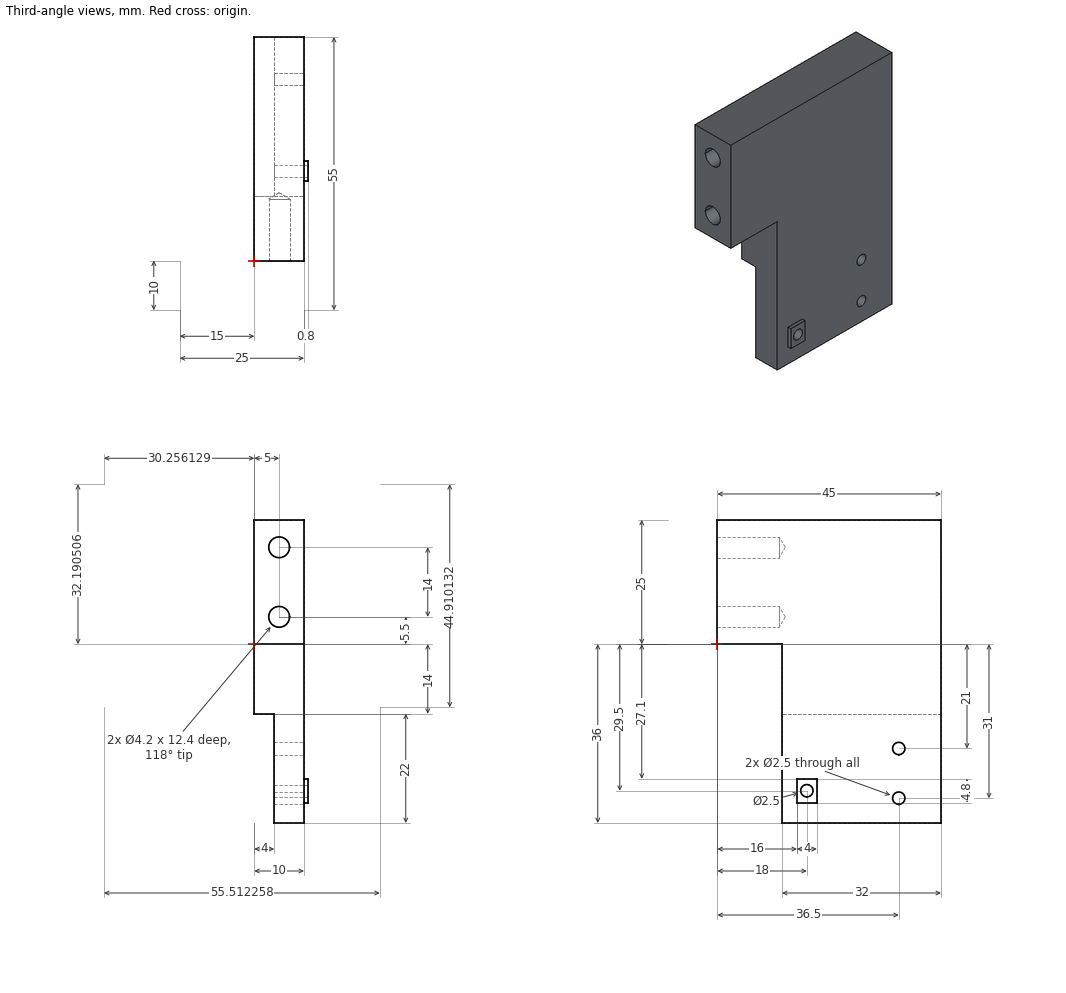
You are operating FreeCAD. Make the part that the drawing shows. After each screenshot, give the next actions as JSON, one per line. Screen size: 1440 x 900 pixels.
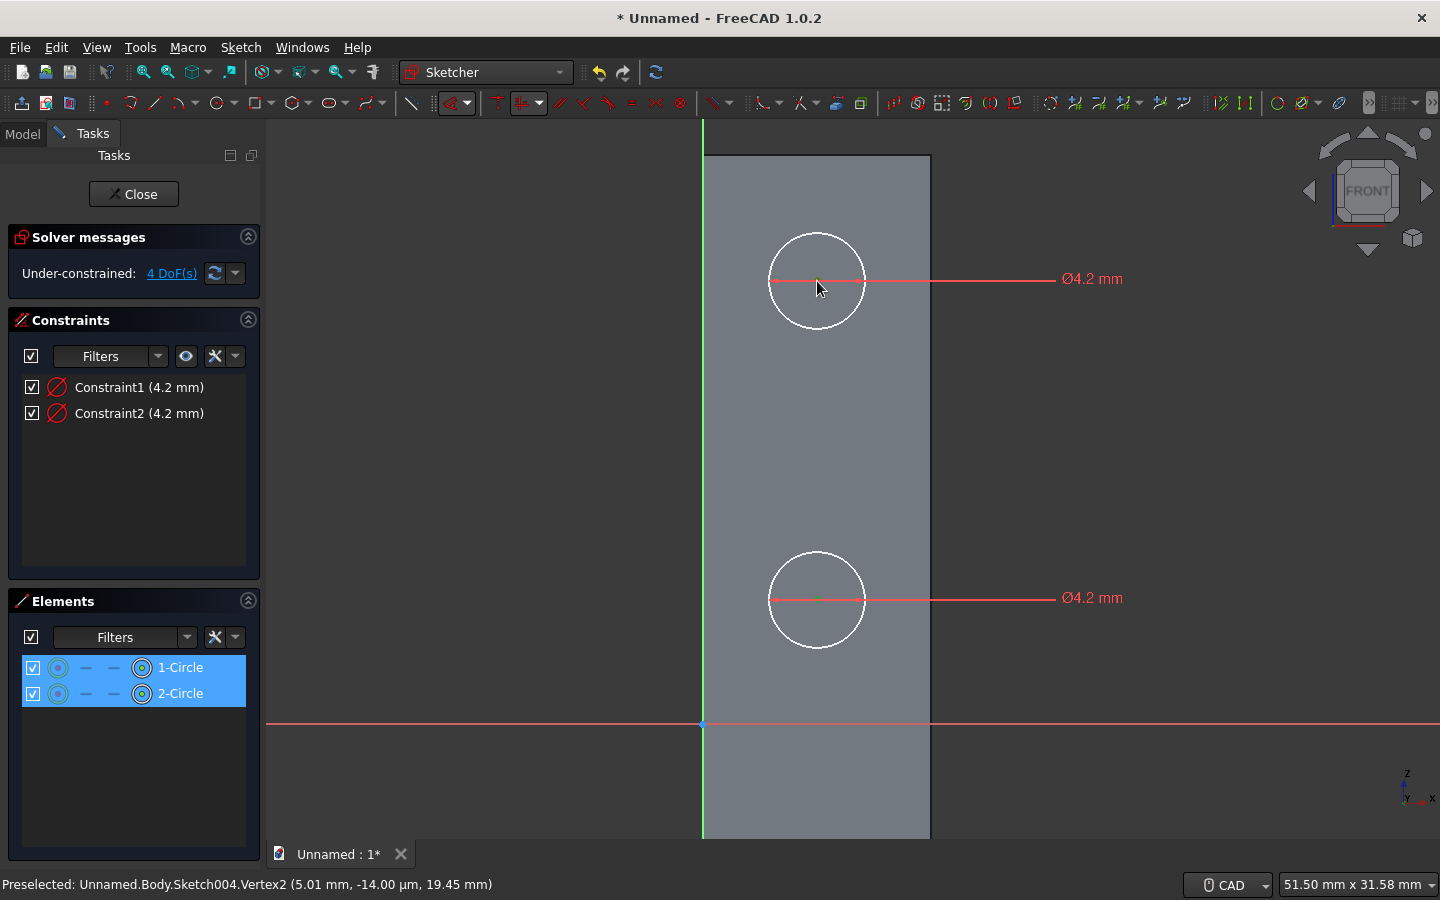
{"action": "key", "text": "v"}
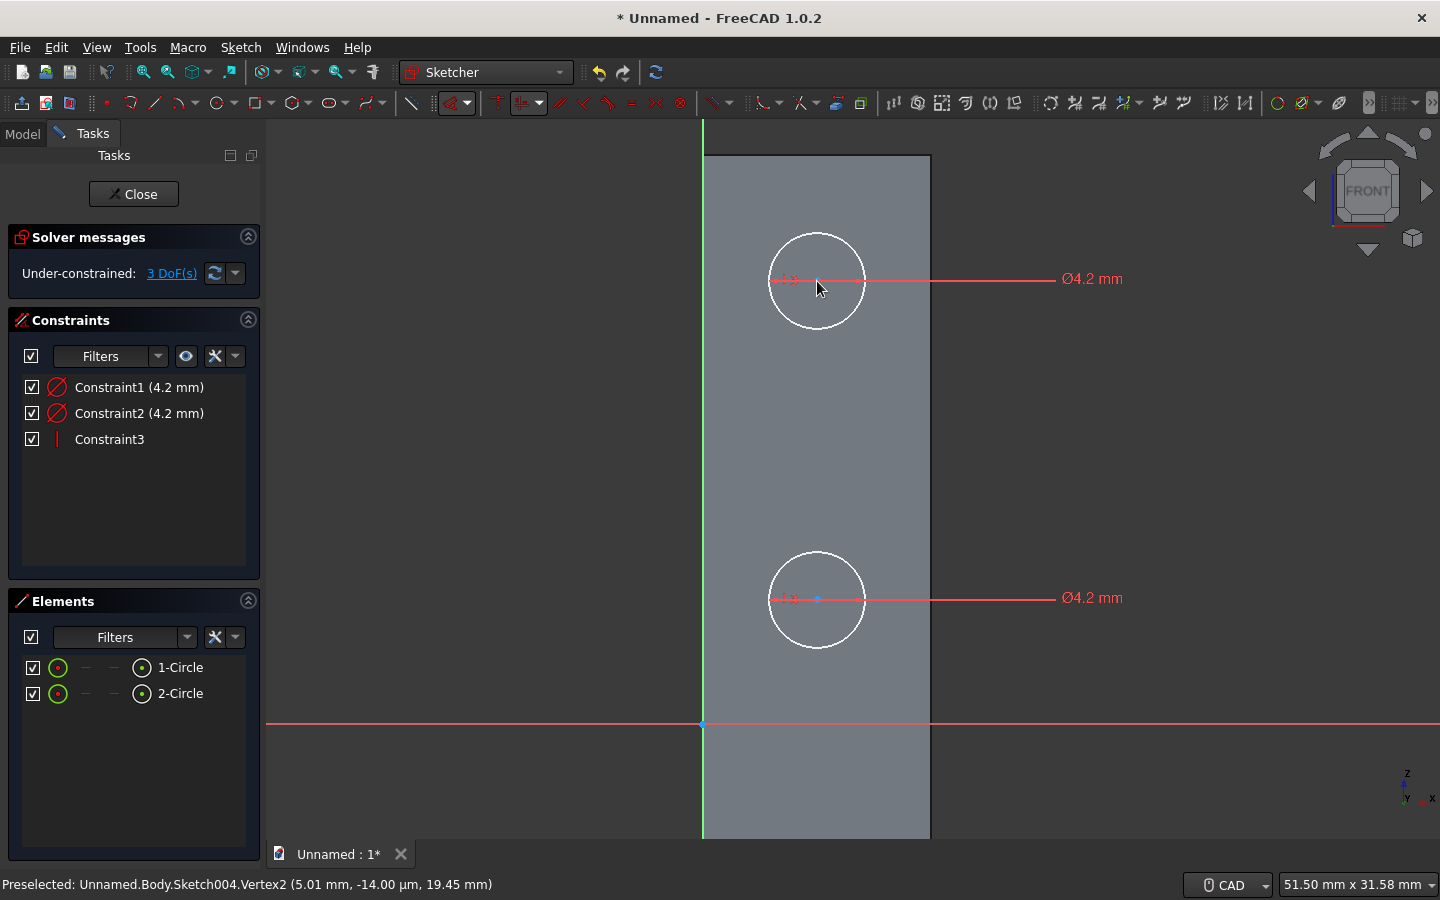
{"action": "left_click", "coordinate": [817, 600]}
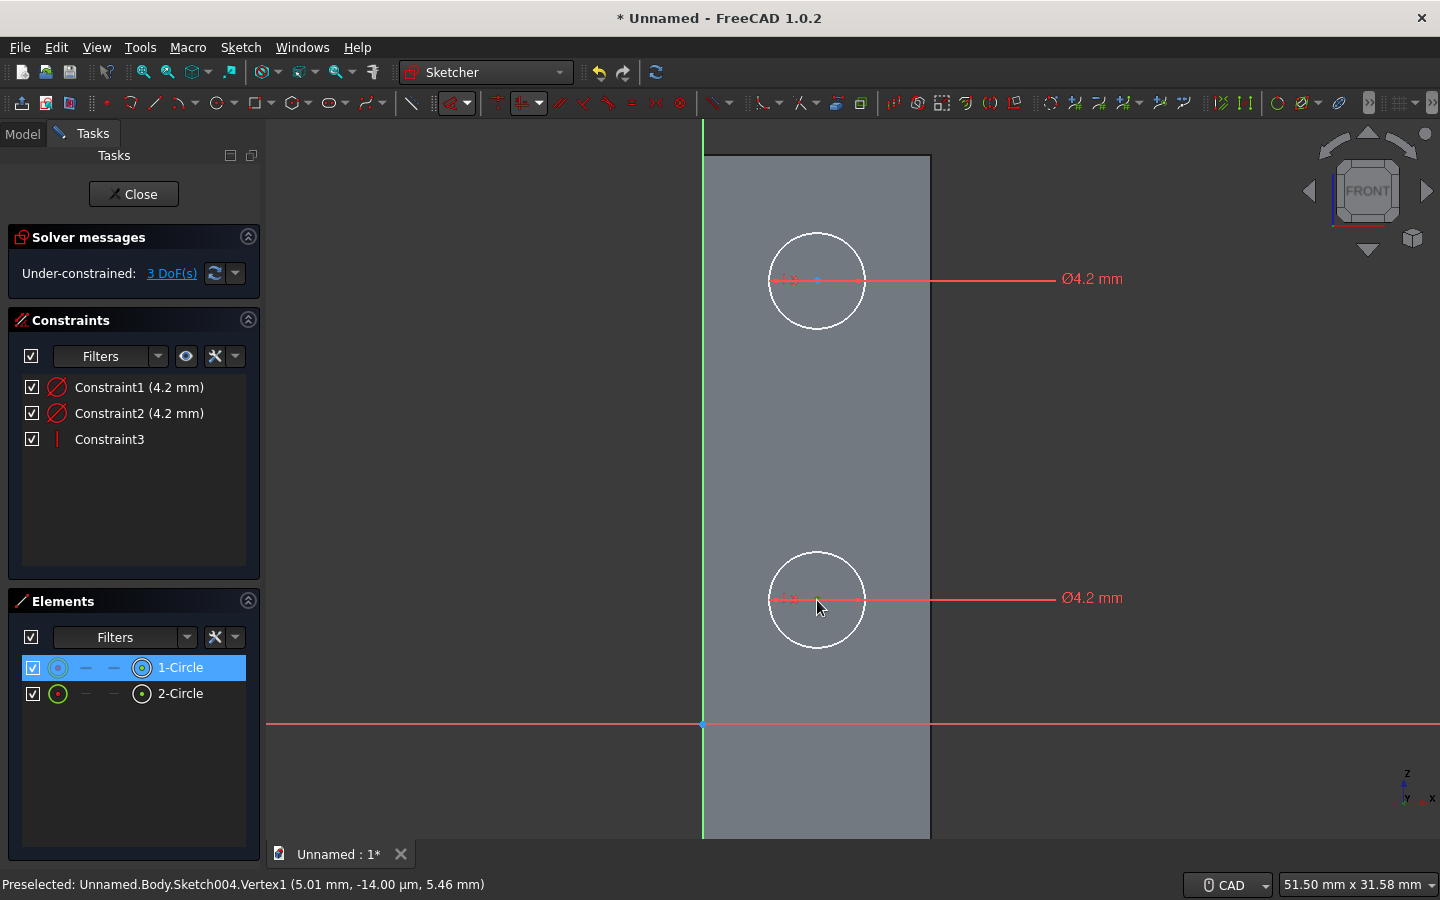
{"action": "key", "text": "l"}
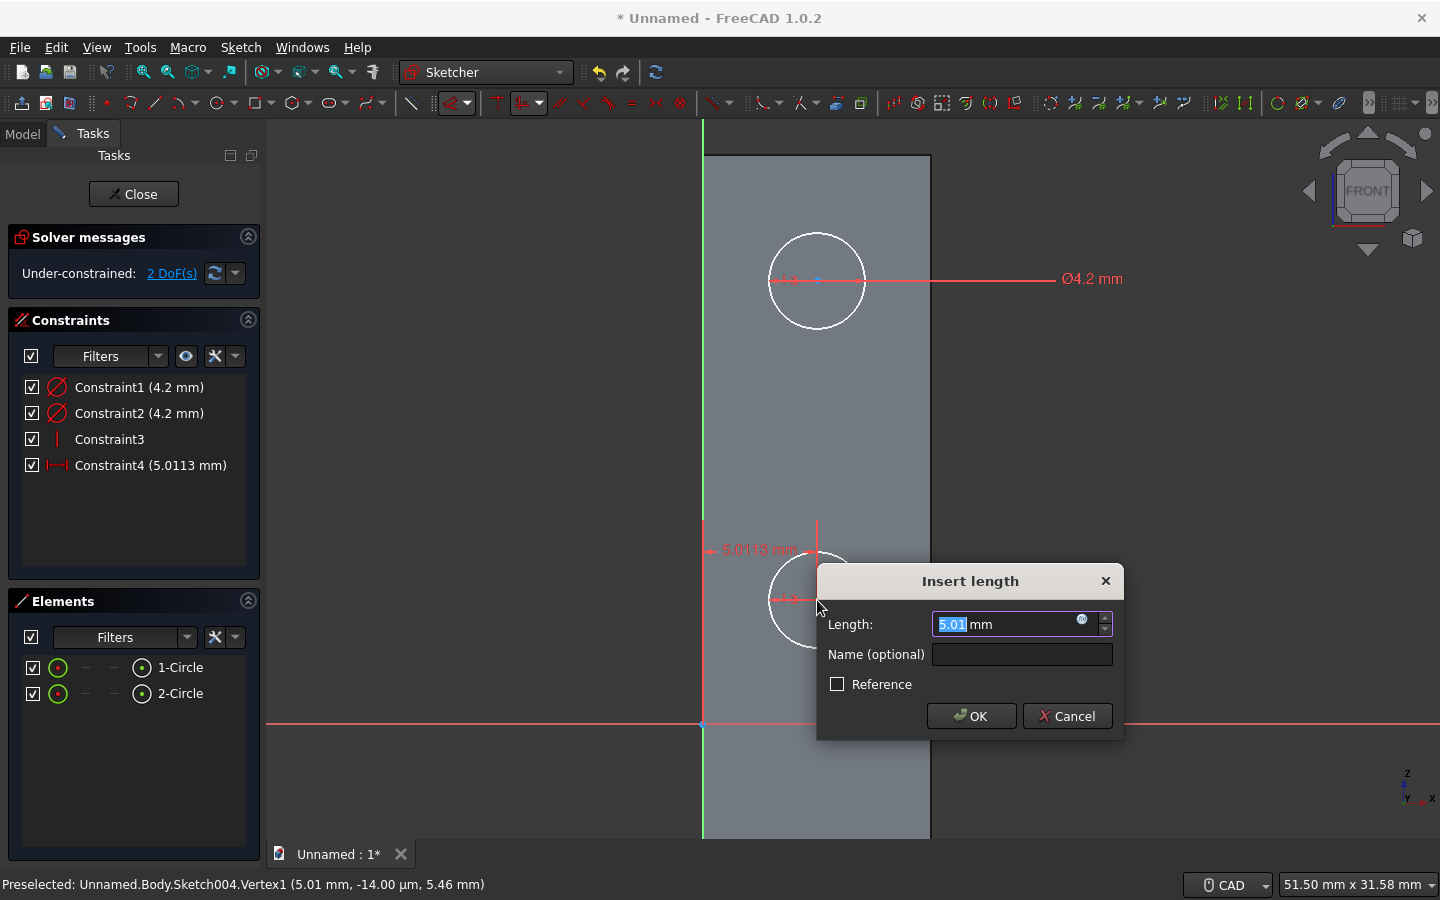
{"action": "type", "text": "5"}
{"action": "key", "text": "Return"}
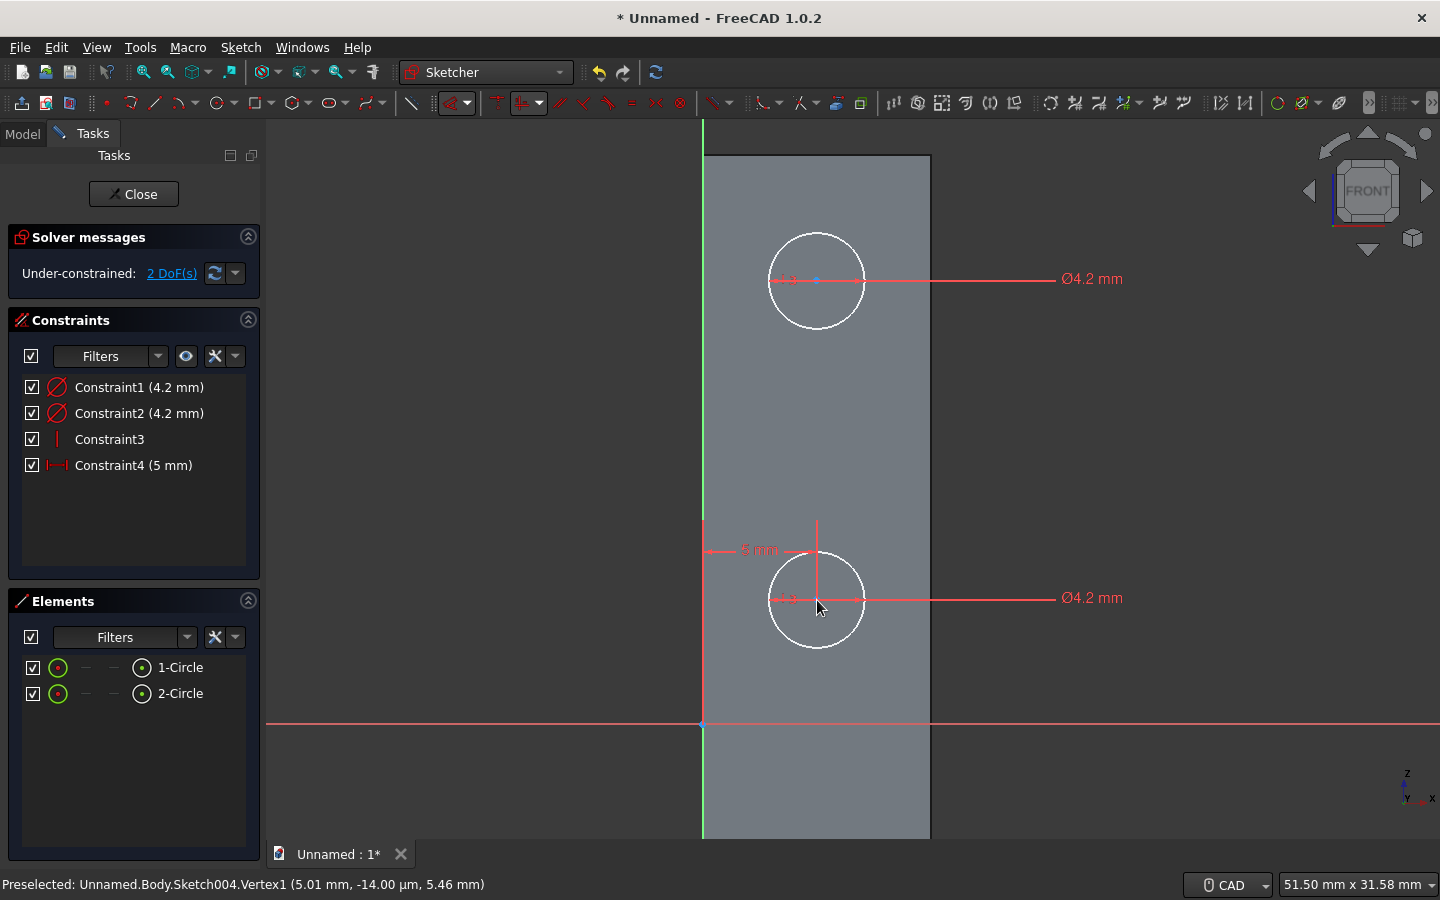
{"action": "left_click", "coordinate": [817, 600]}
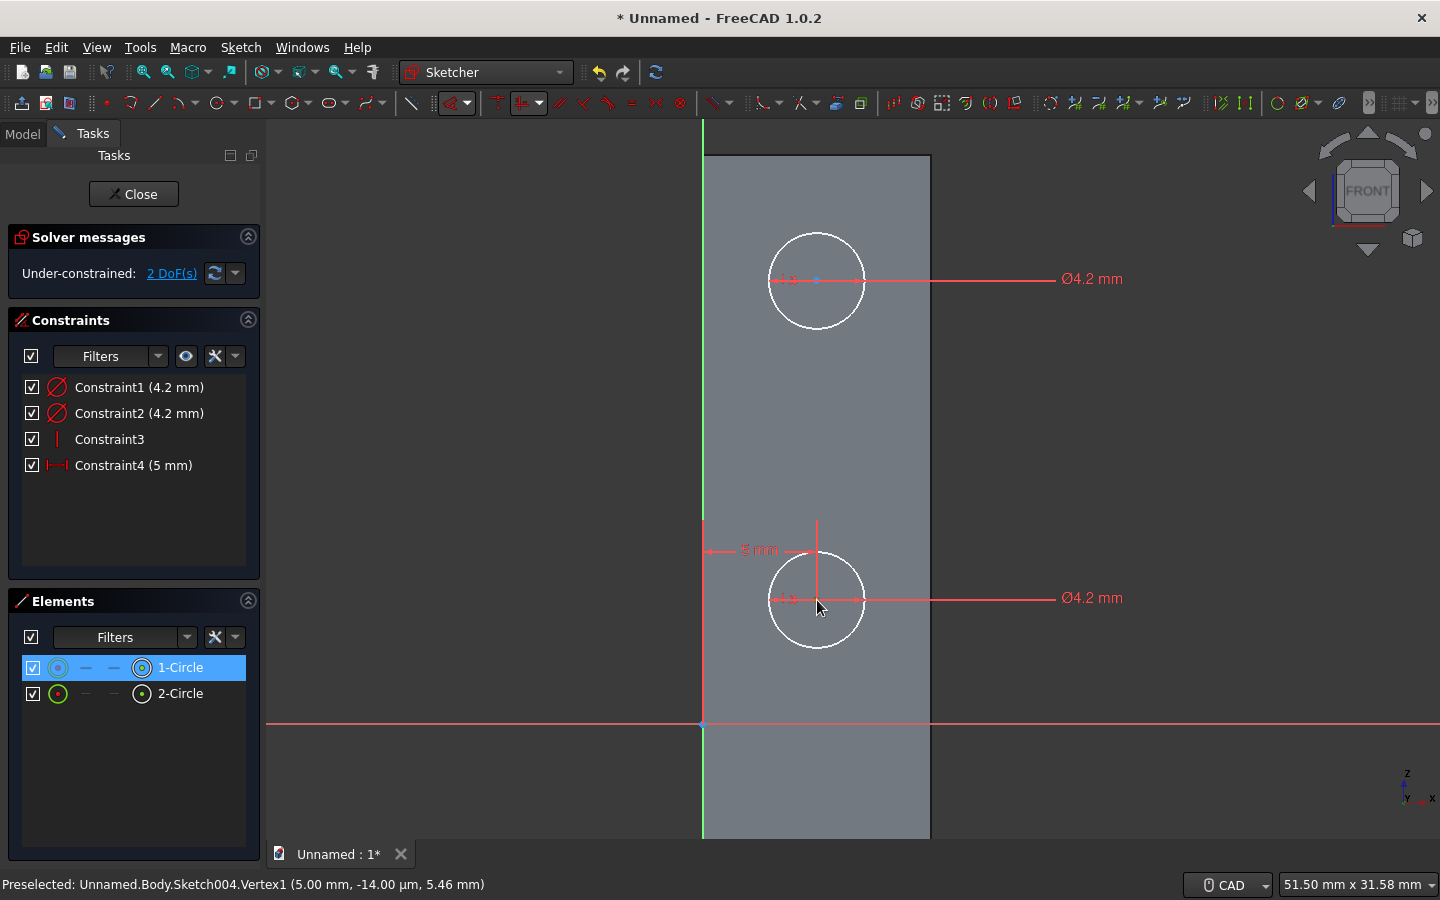
{"action": "left_click", "coordinate": [470, 104]}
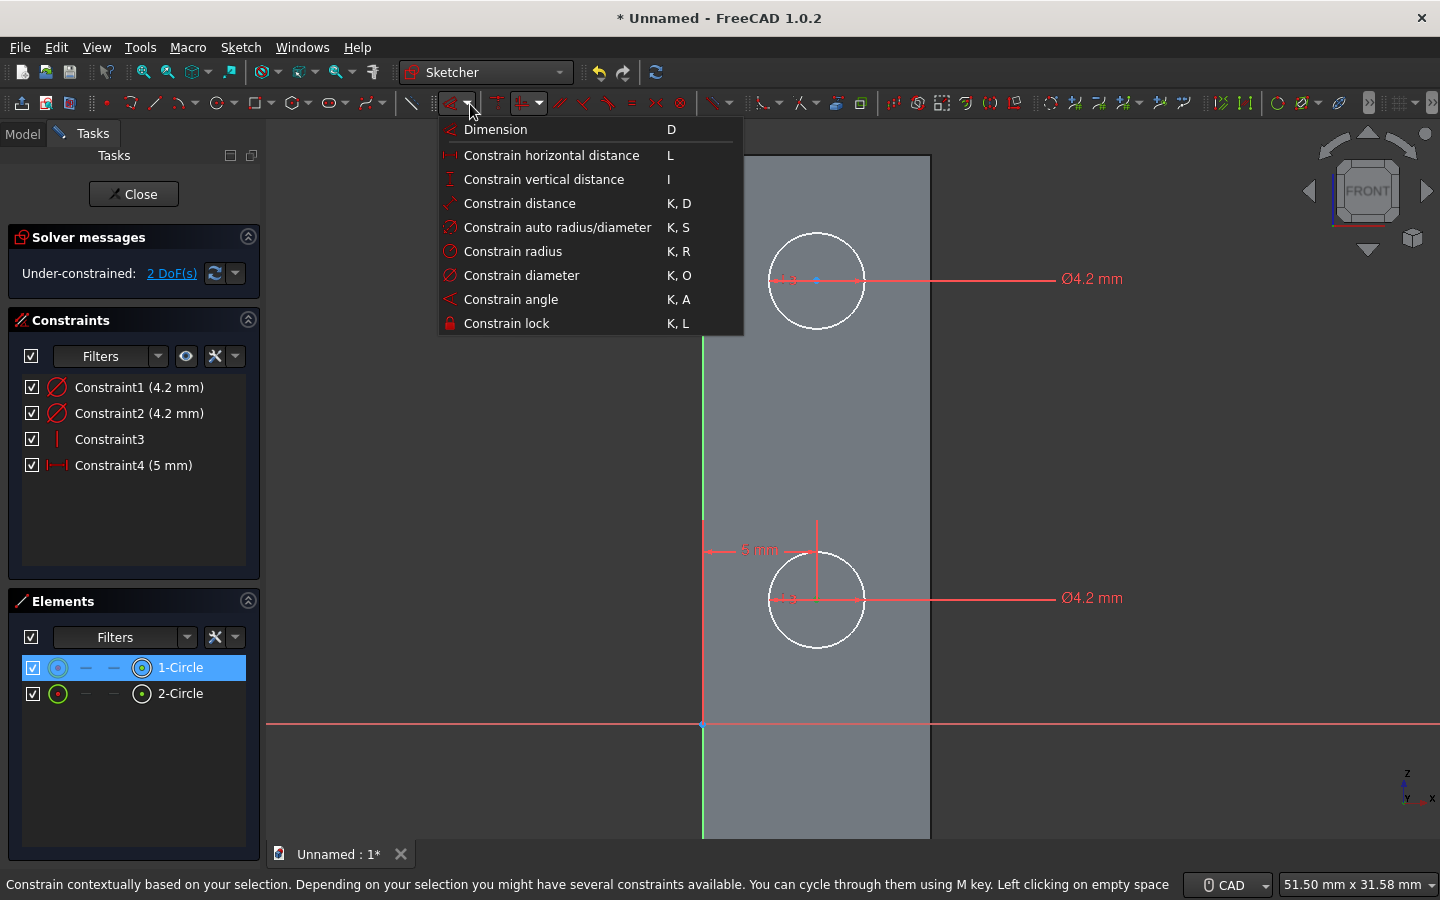
{"action": "left_click", "coordinate": [591, 179]}